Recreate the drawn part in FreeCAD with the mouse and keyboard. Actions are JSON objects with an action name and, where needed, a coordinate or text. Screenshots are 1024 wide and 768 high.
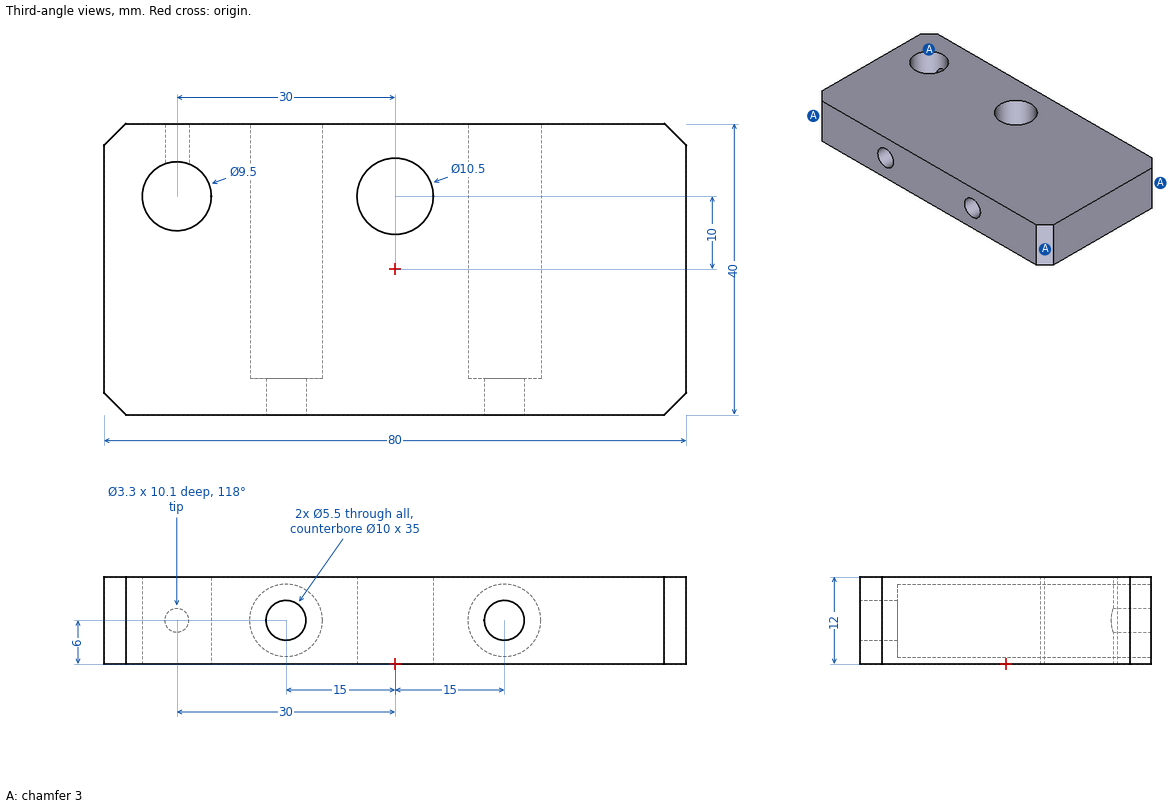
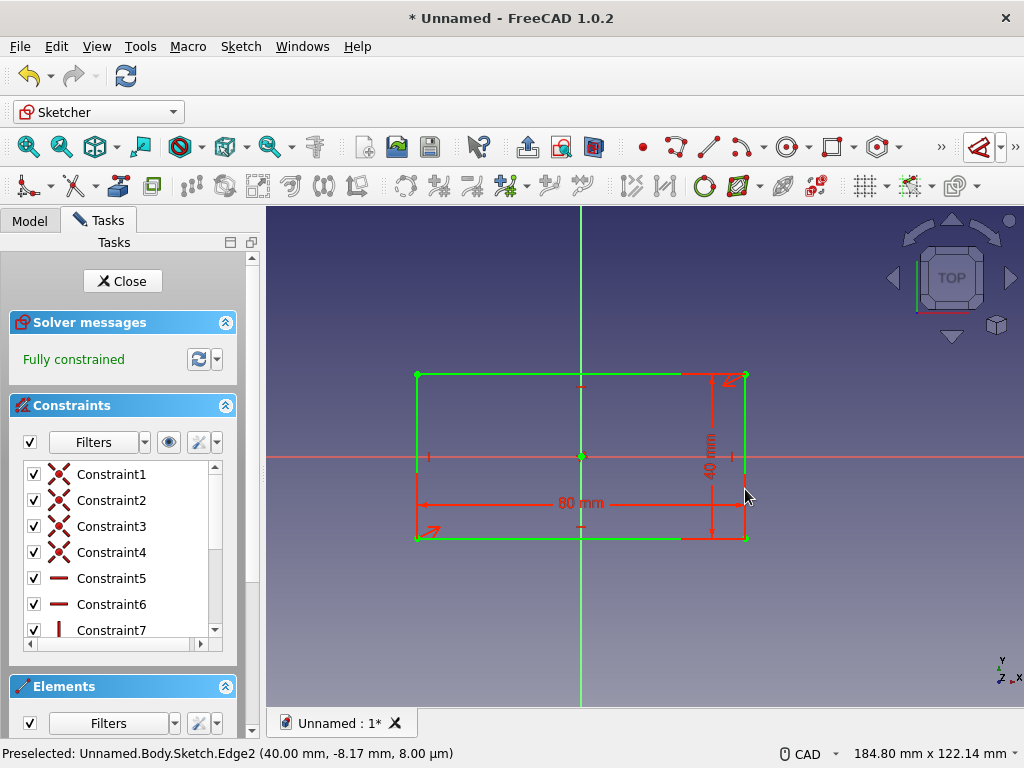
{"action": "left_click", "coordinate": [123, 281]}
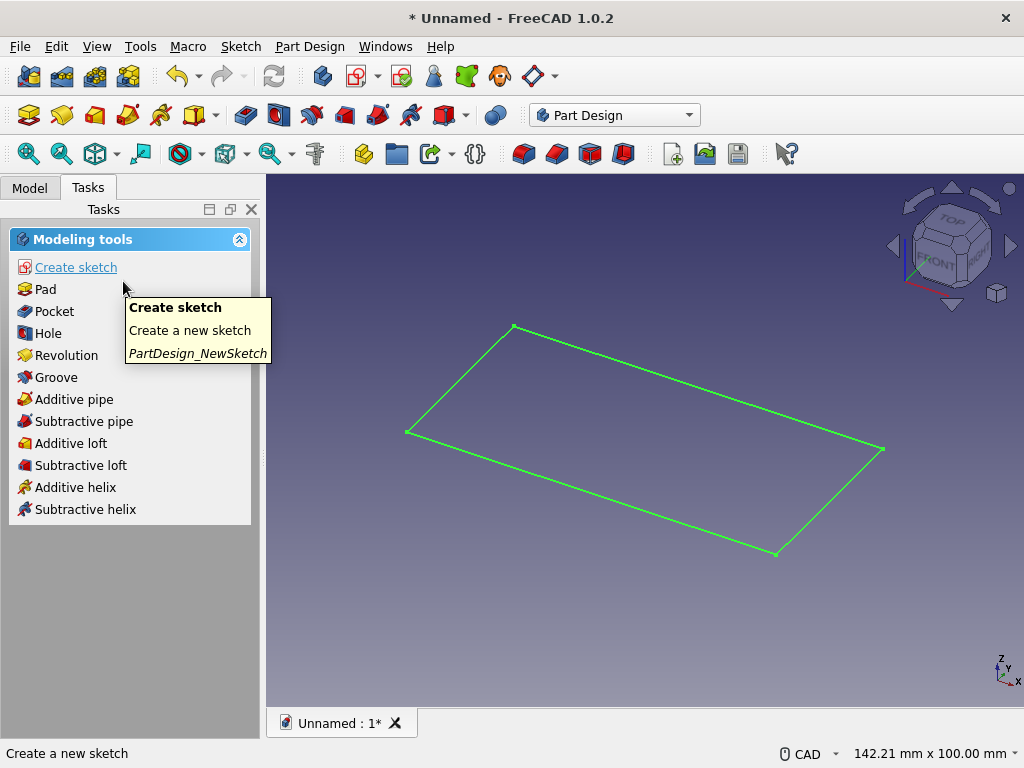
{"action": "left_click", "coordinate": [29, 116]}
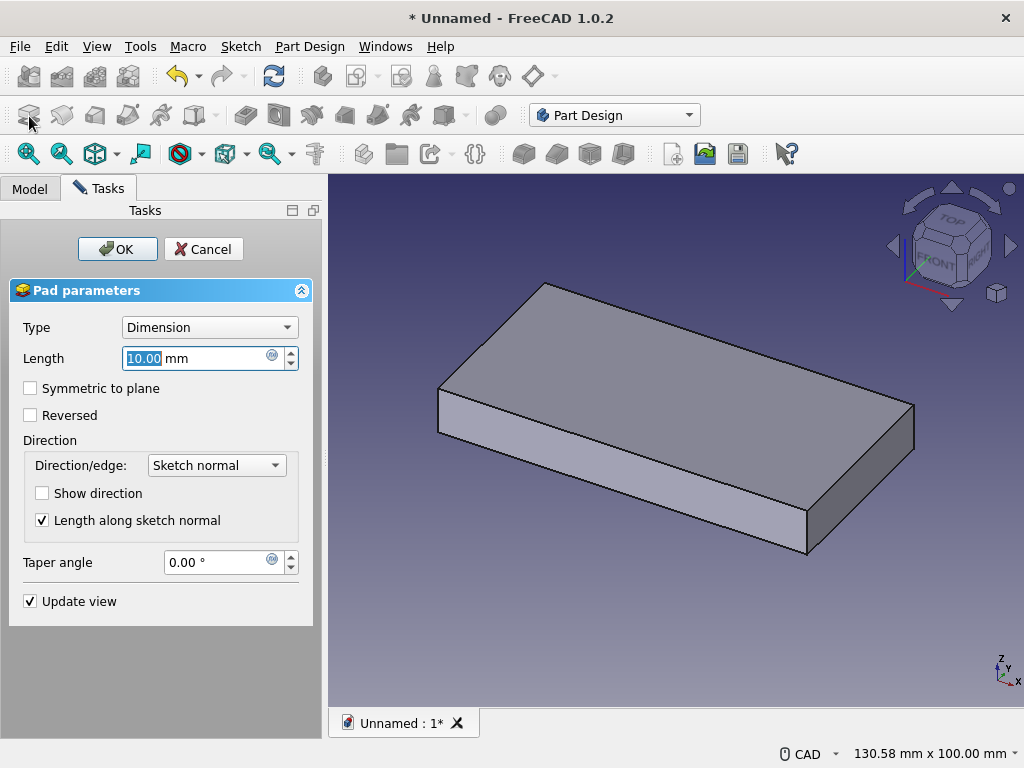
{"action": "type", "text": "12"}
{"action": "key", "text": "Tab"}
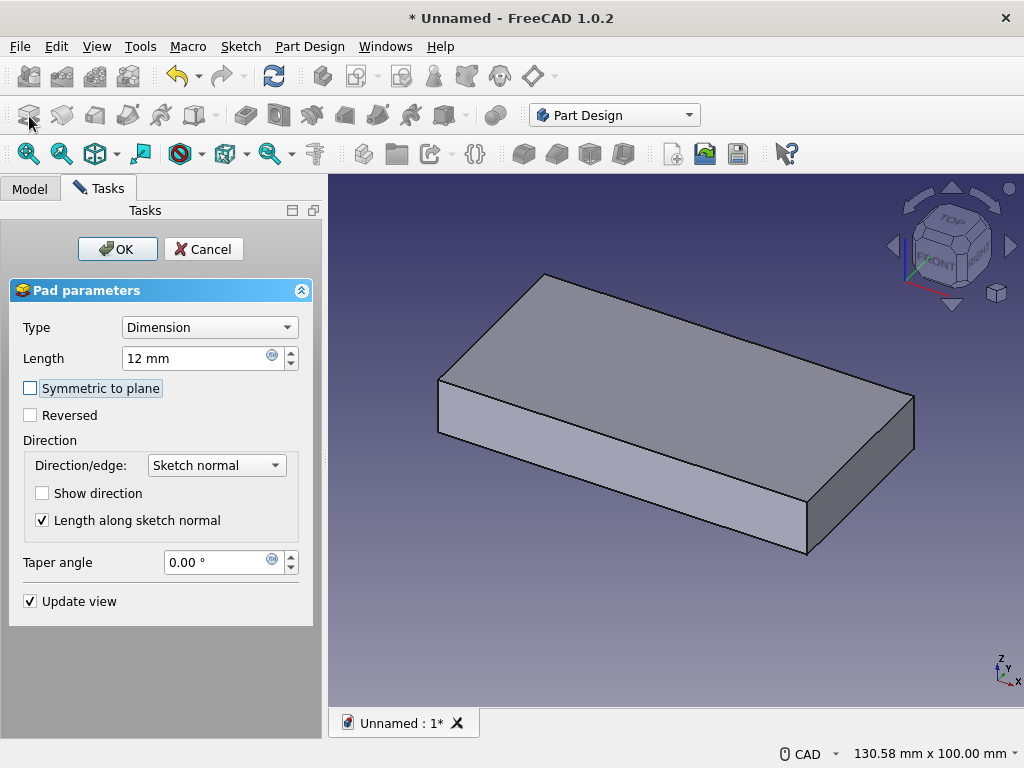
{"action": "left_click", "coordinate": [118, 249]}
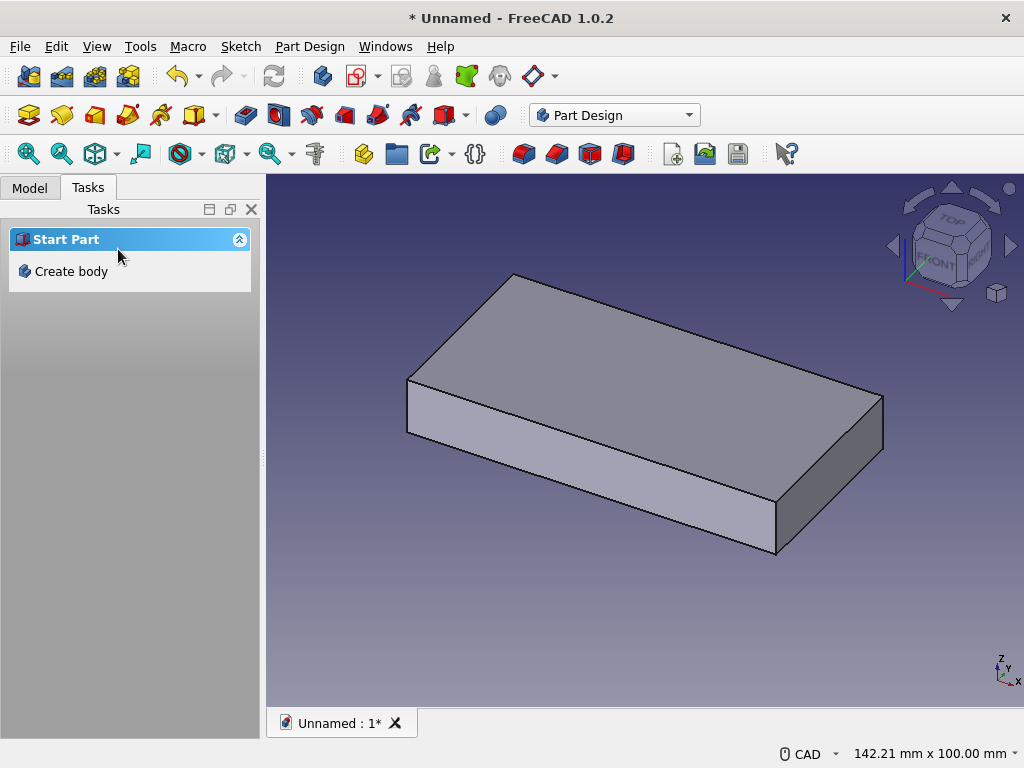
{"action": "left_click", "coordinate": [698, 405]}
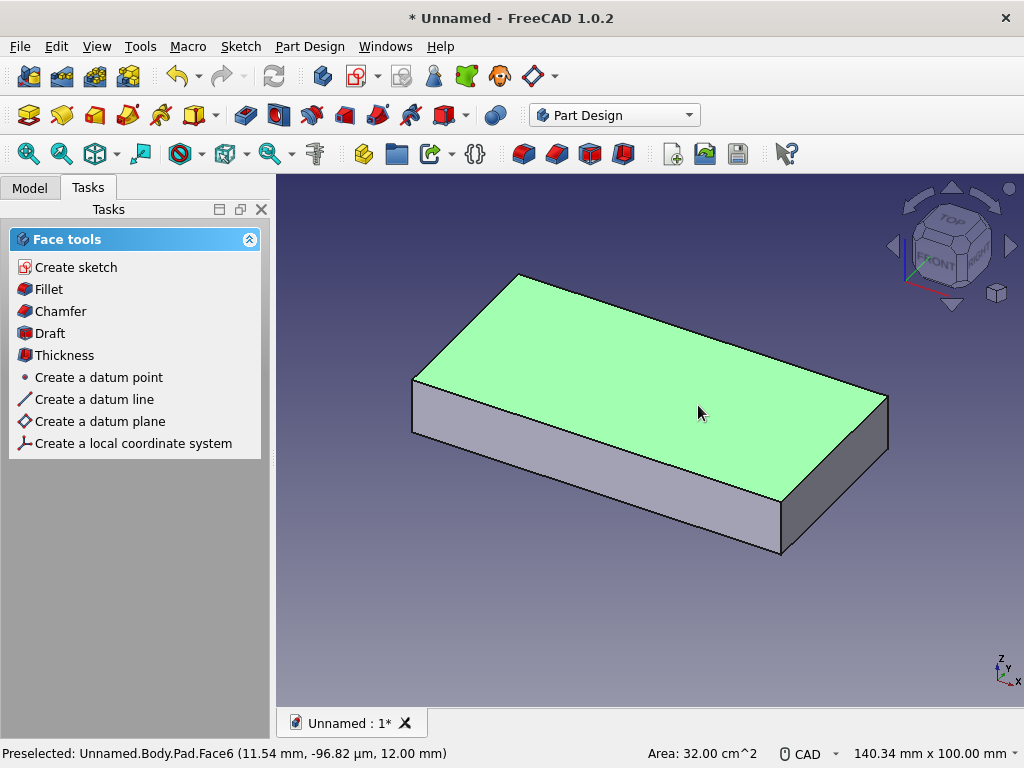
{"action": "left_click", "coordinate": [356, 76]}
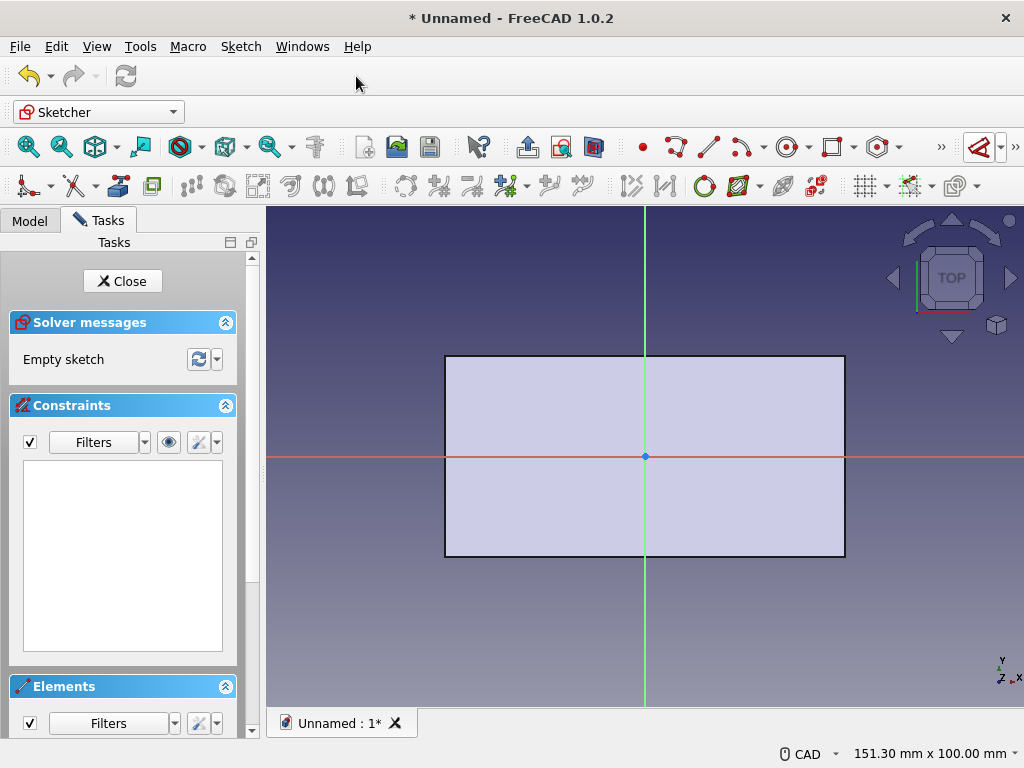
{"action": "scroll", "coordinate": [565, 372], "scroll_direction": "up", "scroll_amount": 3}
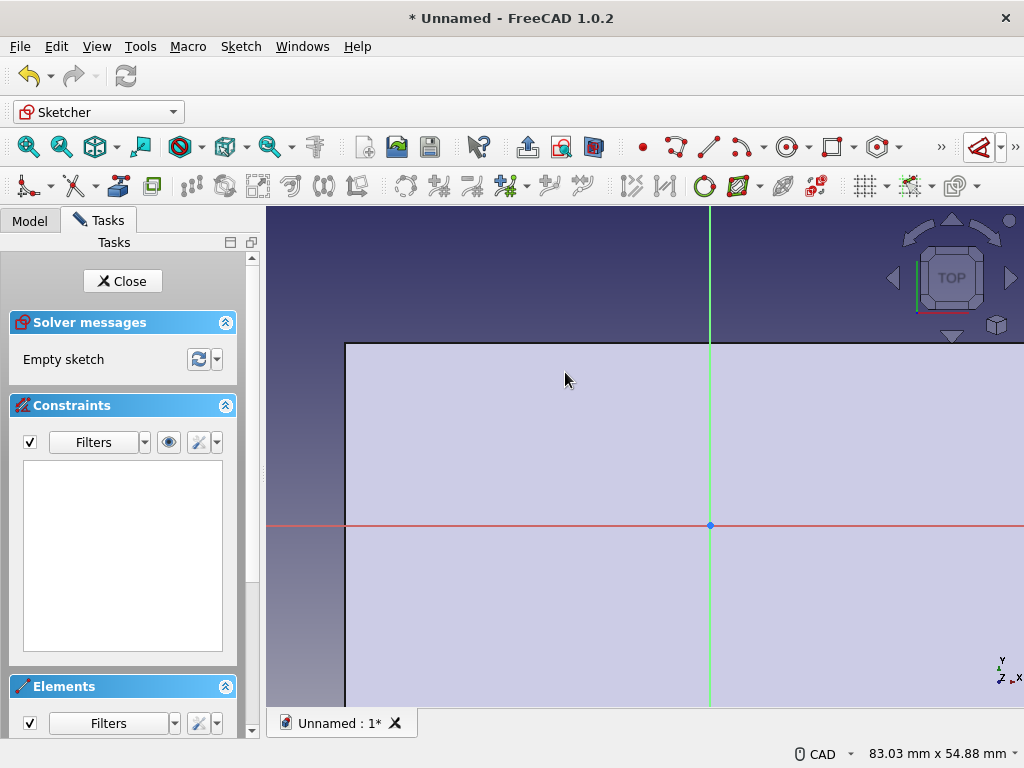
{"action": "left_click", "coordinate": [786, 148]}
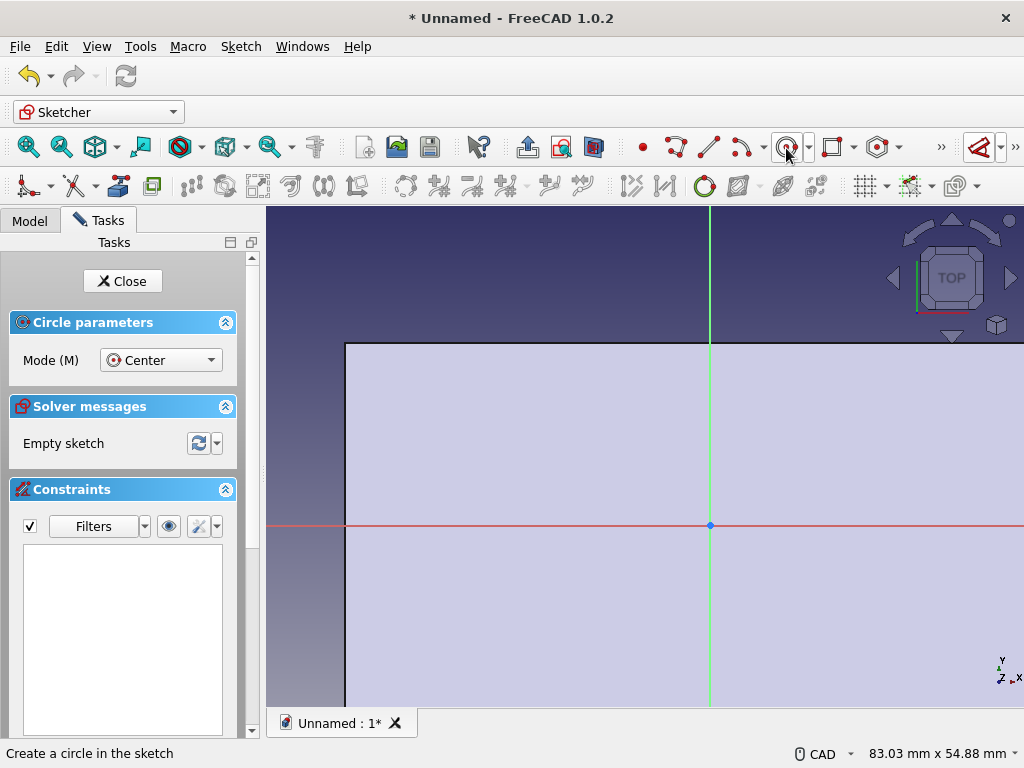
{"action": "left_click", "coordinate": [710, 434]}
{"action": "left_click", "coordinate": [744, 401]}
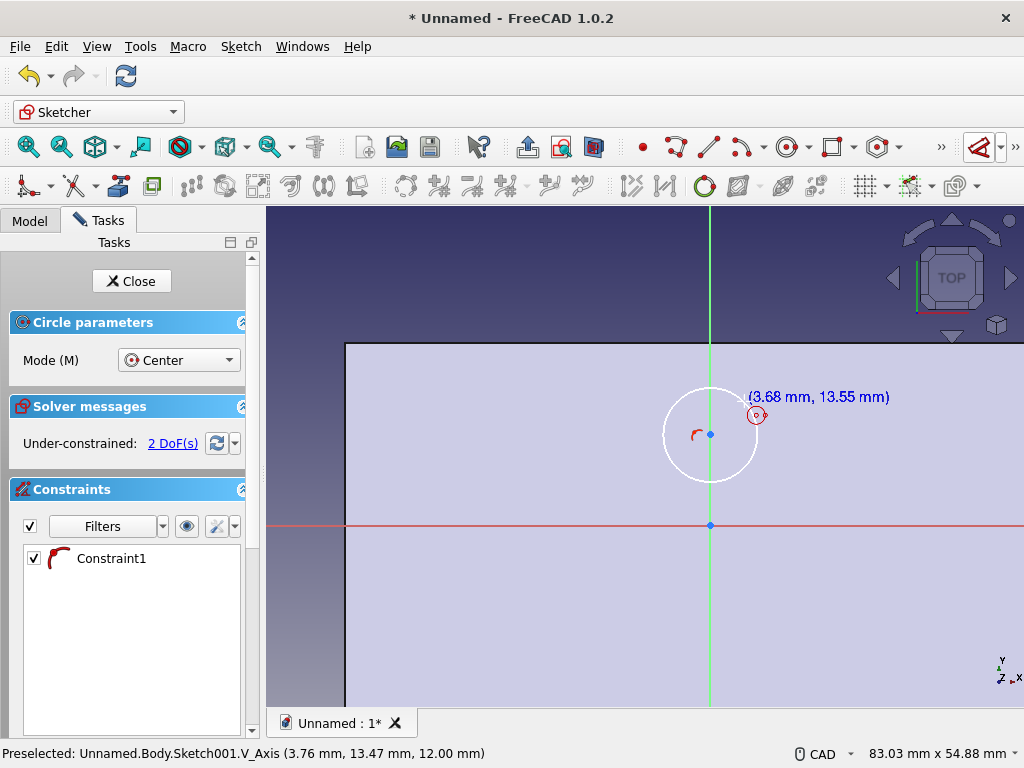
{"action": "left_click", "coordinate": [437, 434]}
{"action": "left_click", "coordinate": [467, 404]}
{"action": "key", "text": "Escape"}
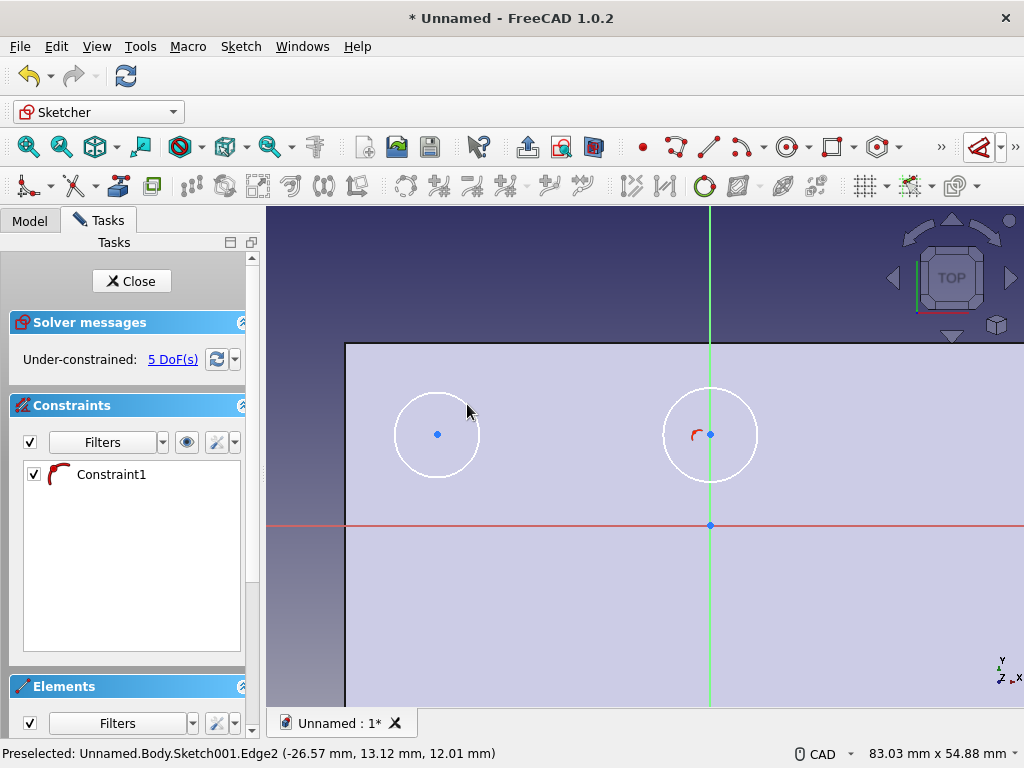
{"action": "left_click", "coordinate": [710, 435]}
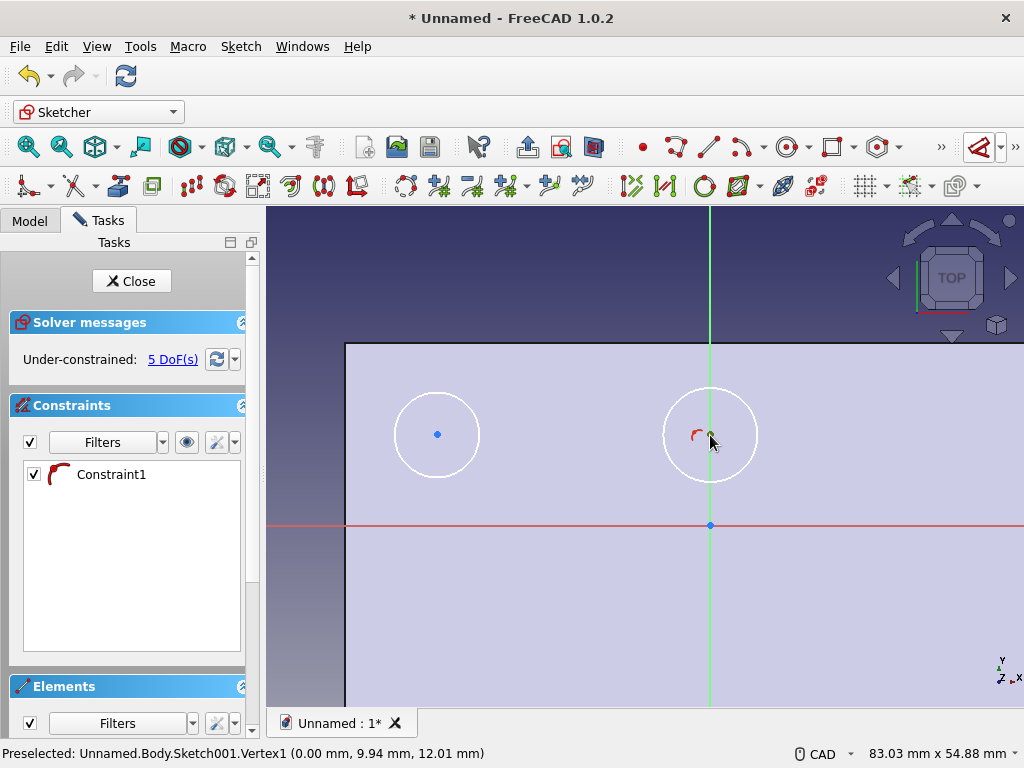
{"action": "left_click", "coordinate": [437, 435]}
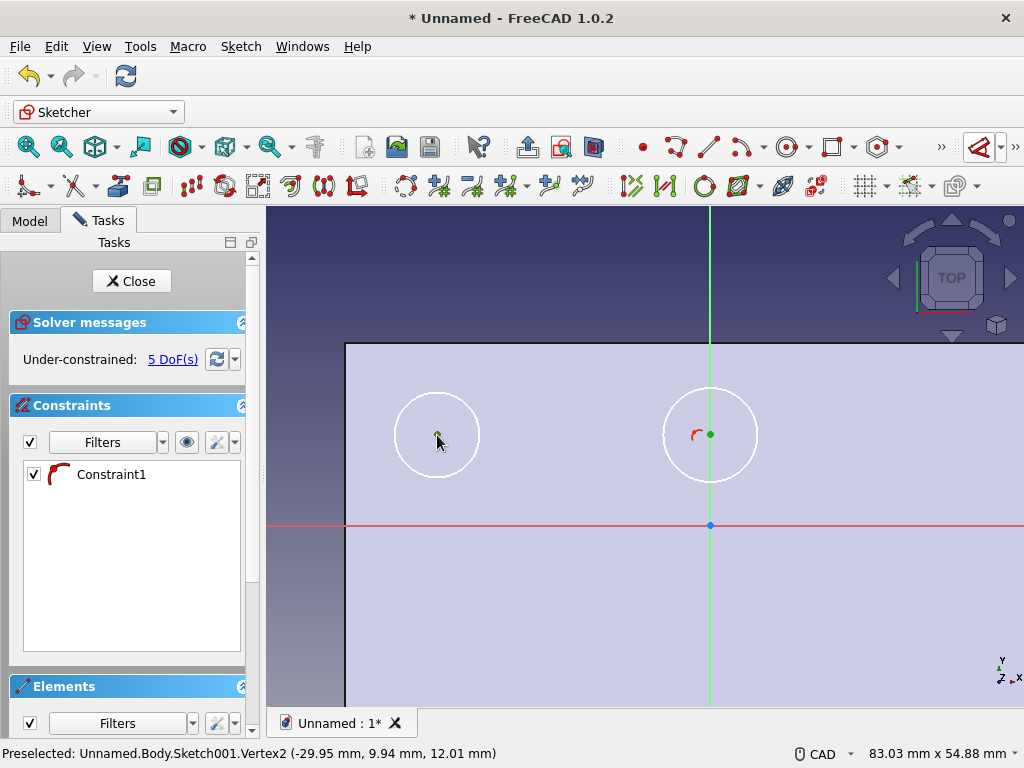
{"action": "key", "text": "h"}